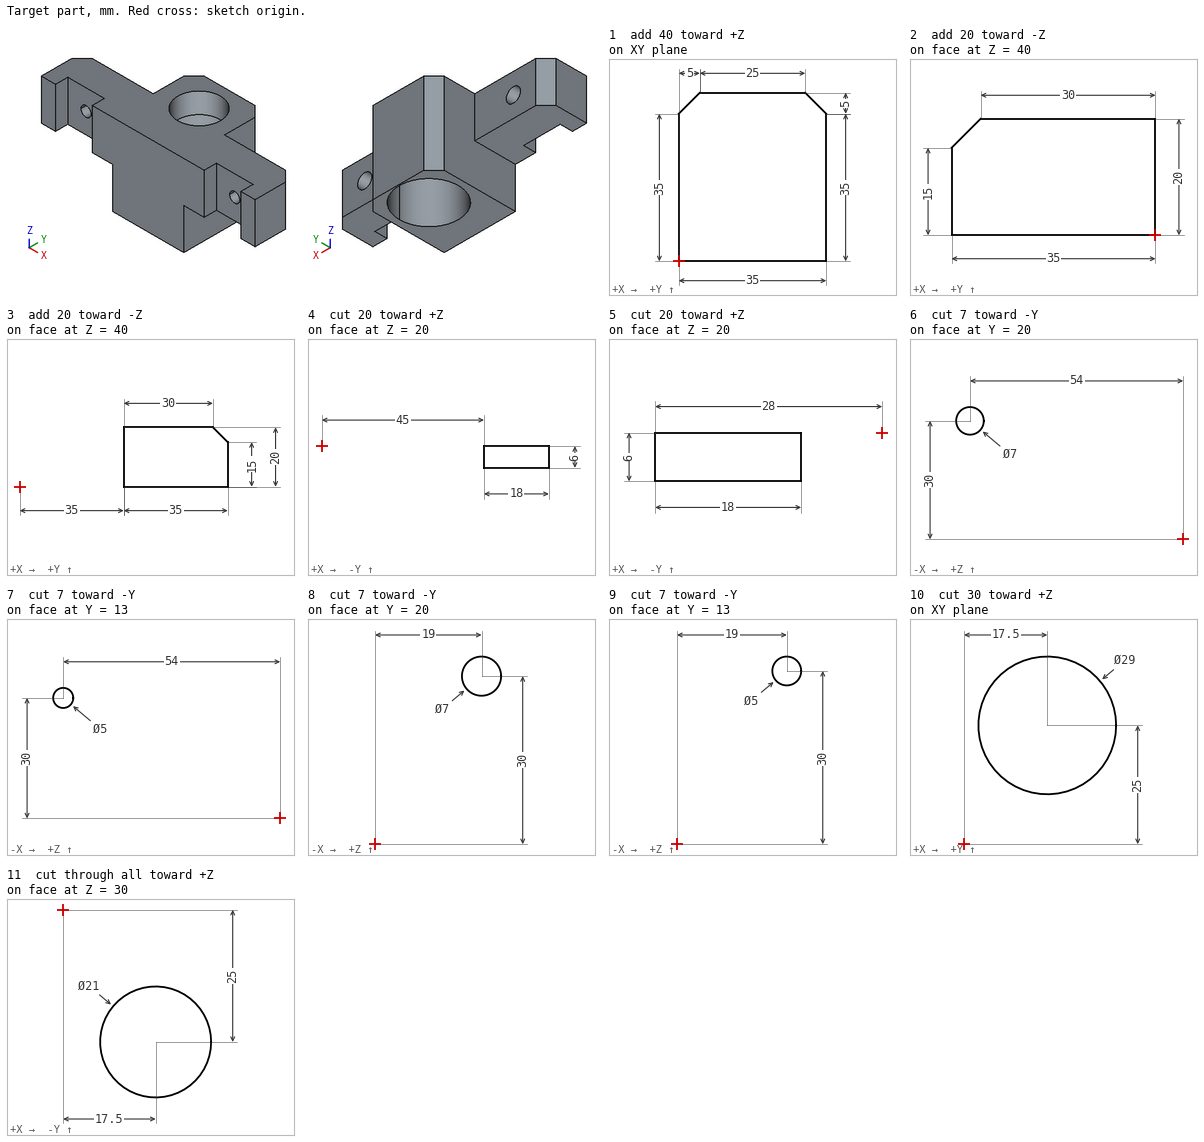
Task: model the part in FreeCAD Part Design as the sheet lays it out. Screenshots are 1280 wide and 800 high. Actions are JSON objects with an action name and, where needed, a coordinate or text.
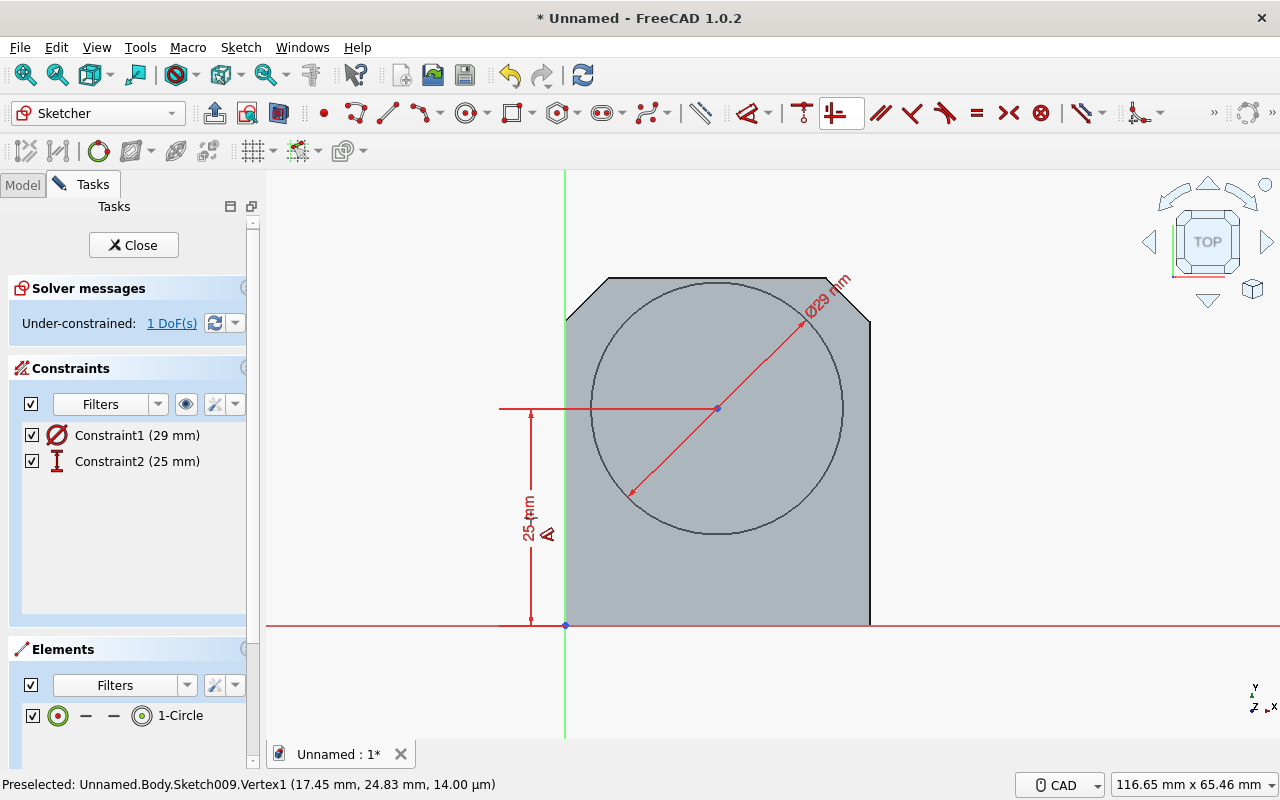
{"action": "left_click", "coordinate": [717, 409]}
{"action": "left_click", "coordinate": [641, 660]}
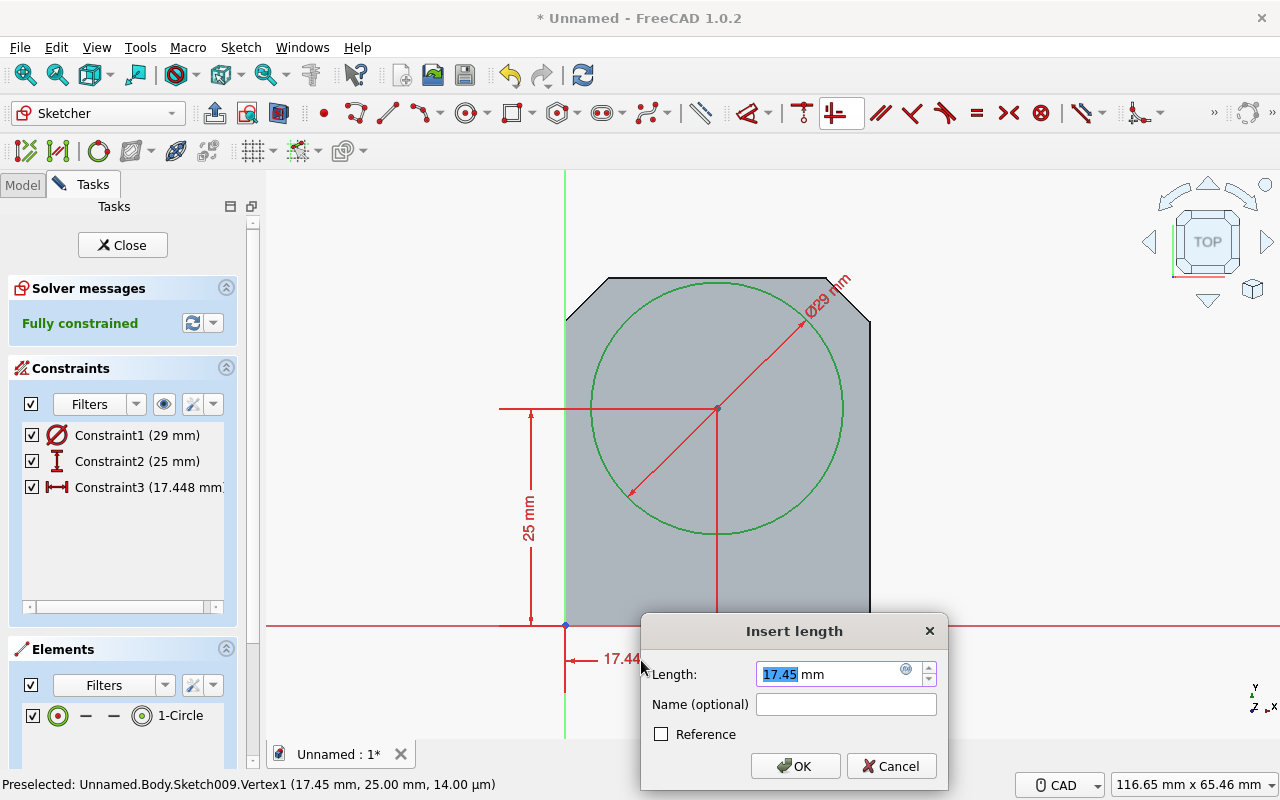
{"action": "type", "text": "17.5"}
{"action": "key", "text": "Return"}
{"action": "key", "text": "Escape"}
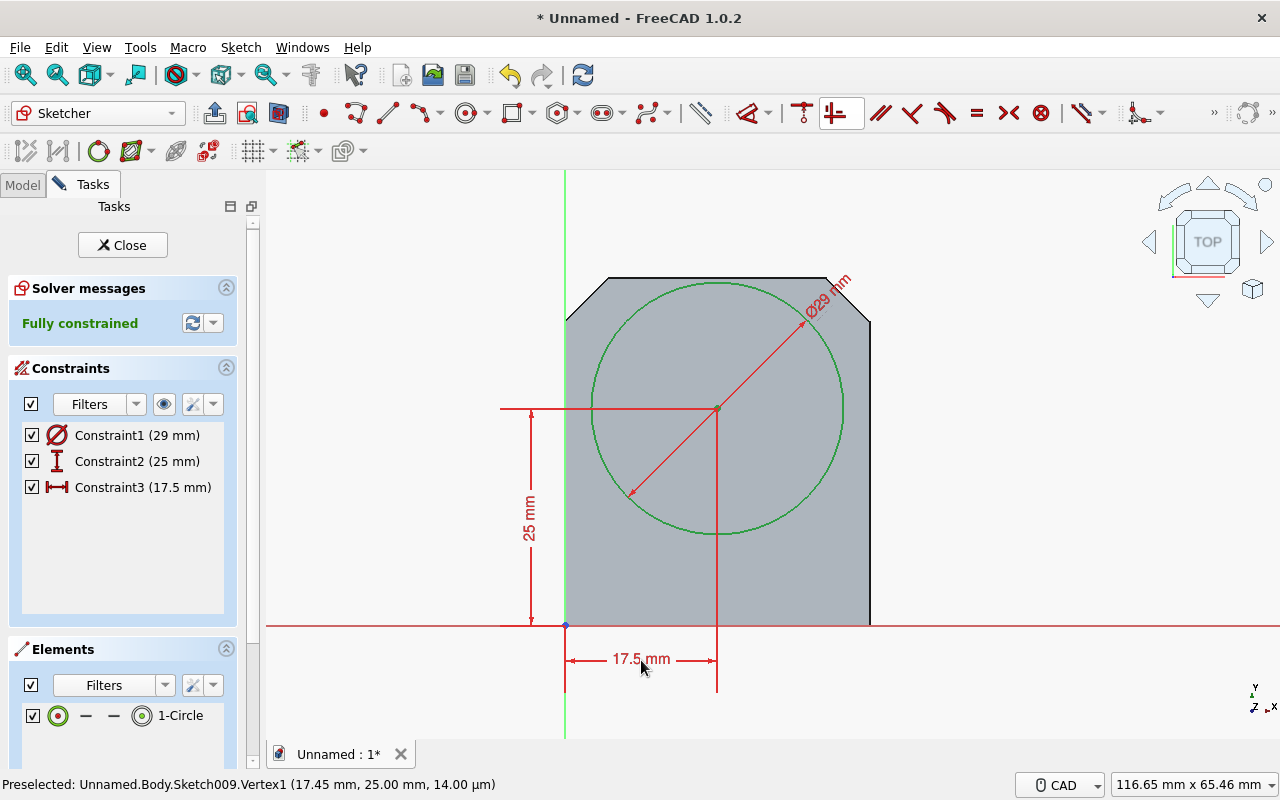
{"action": "left_click", "coordinate": [123, 245]}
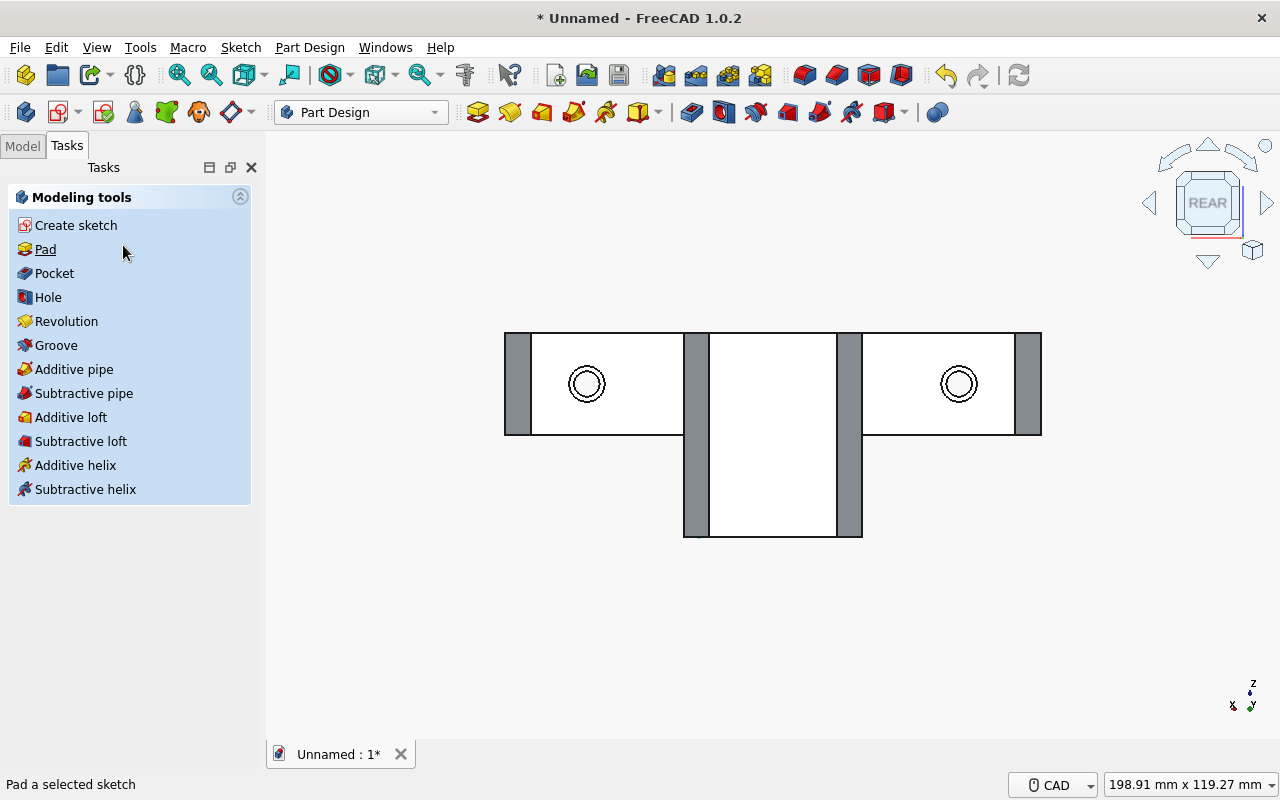
{"action": "left_click", "coordinate": [692, 112]}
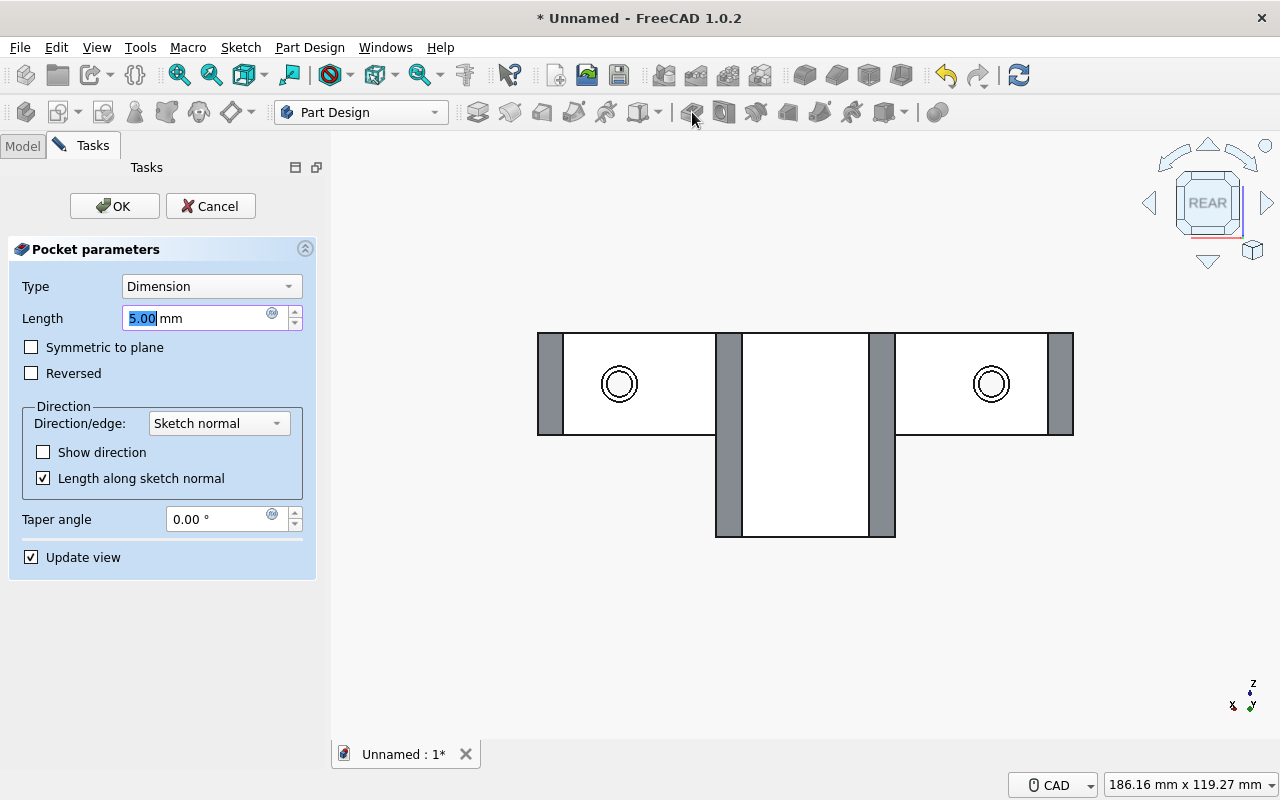
{"action": "type", "text": "30"}
{"action": "key", "text": "Tab"}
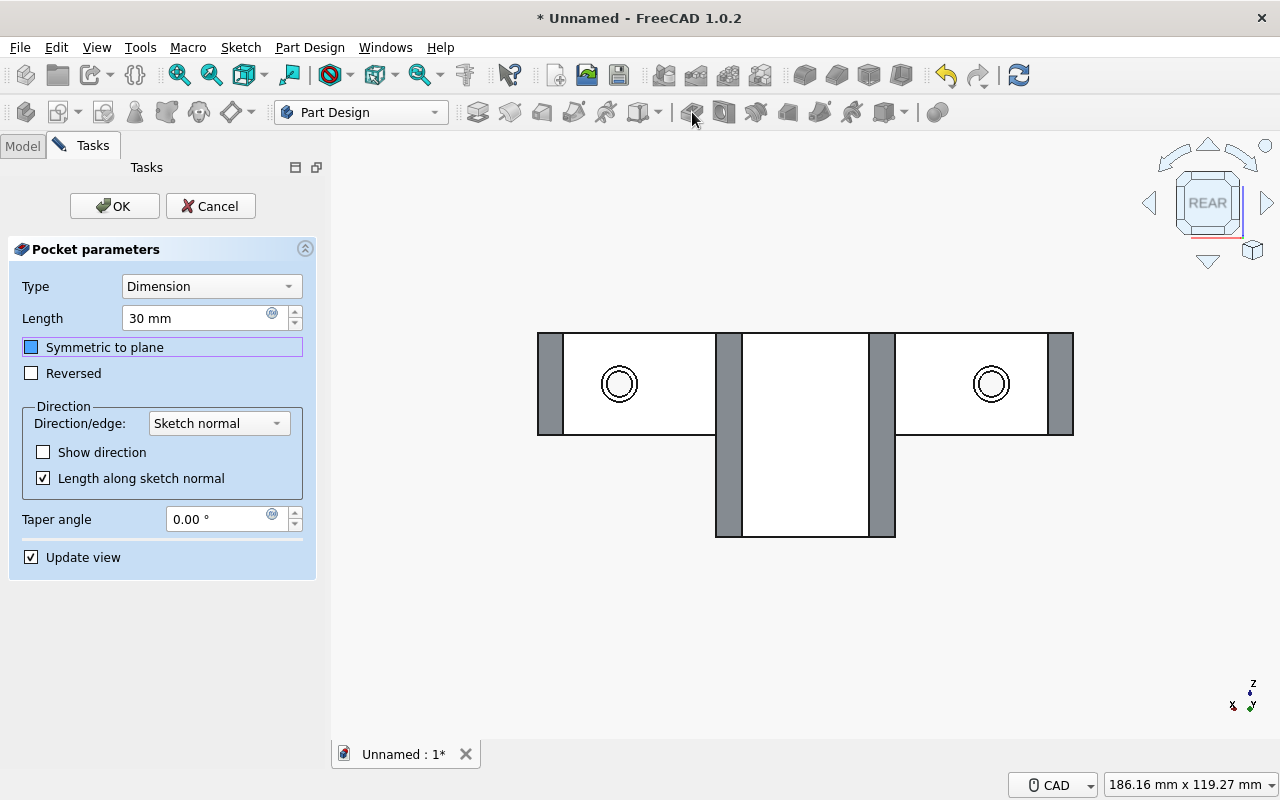
{"action": "left_click", "coordinate": [30, 373]}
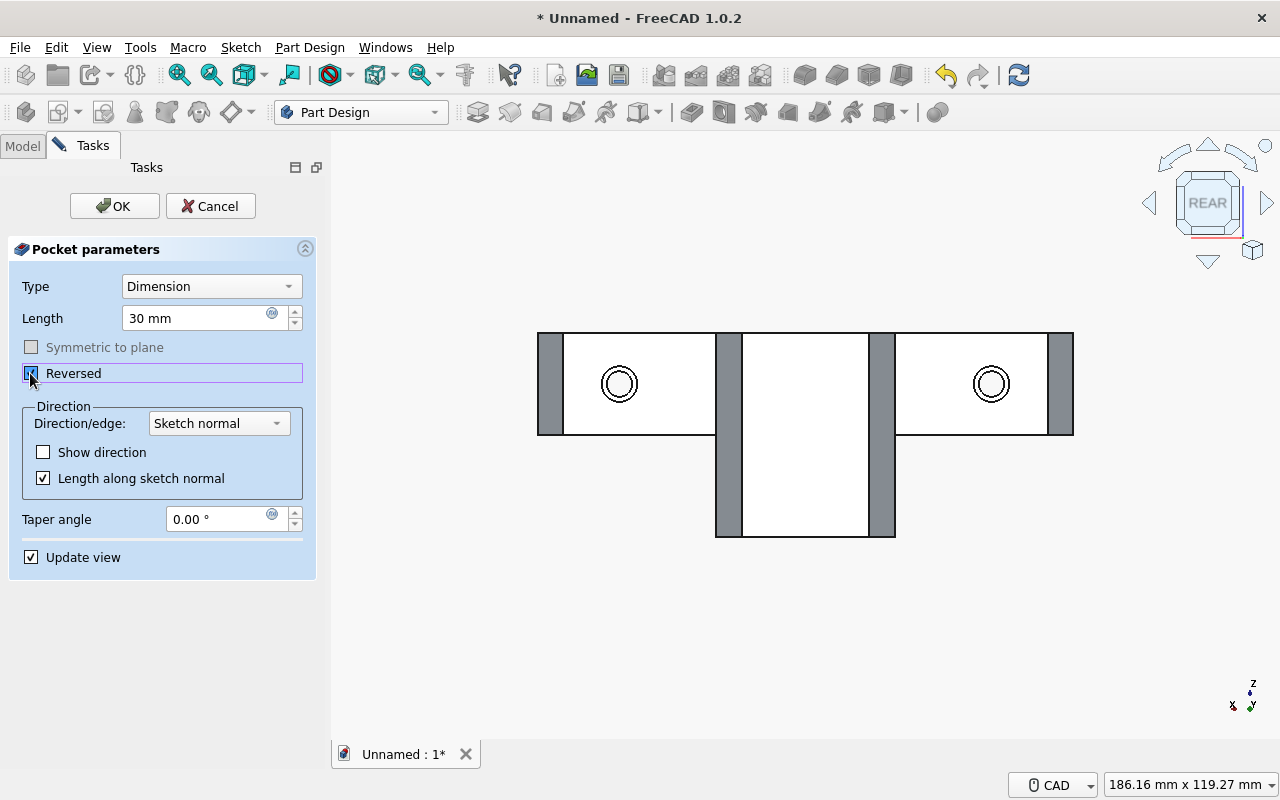
{"action": "left_click", "coordinate": [115, 206]}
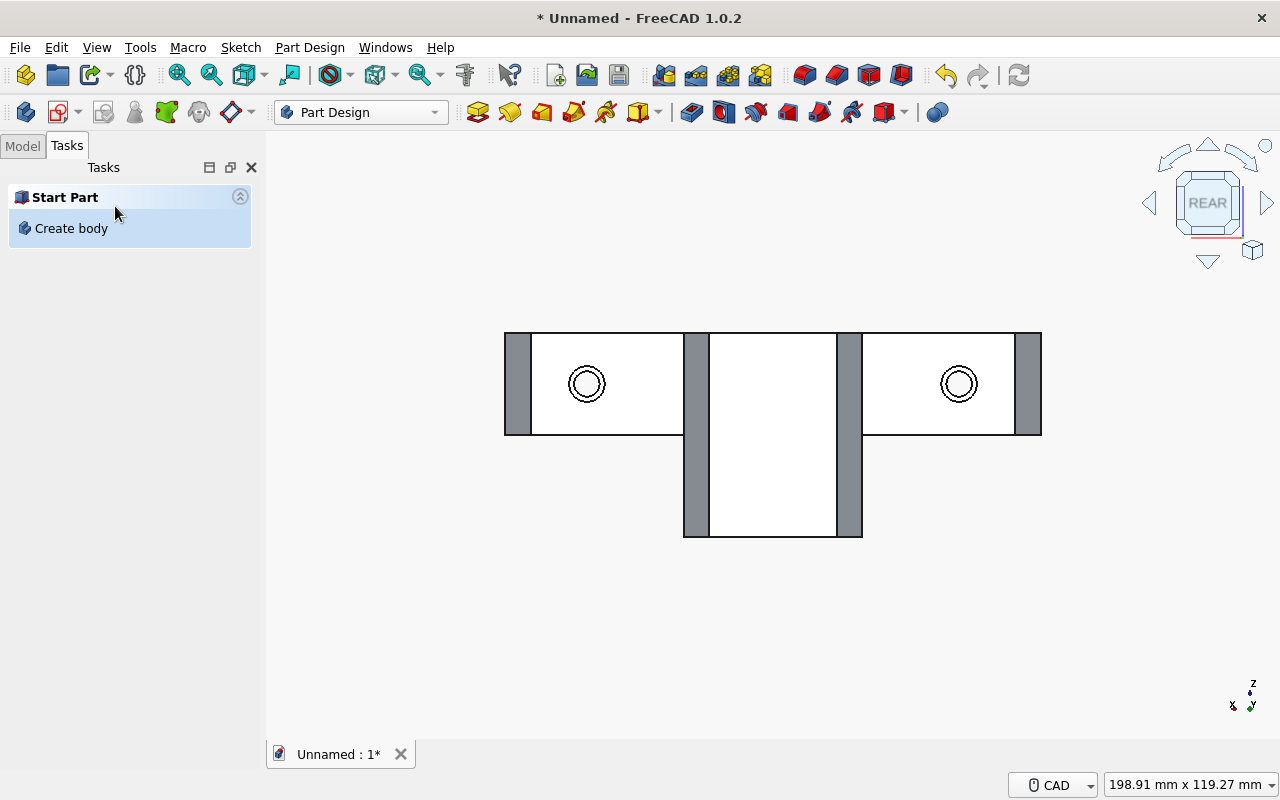
{"action": "key", "text": "5"}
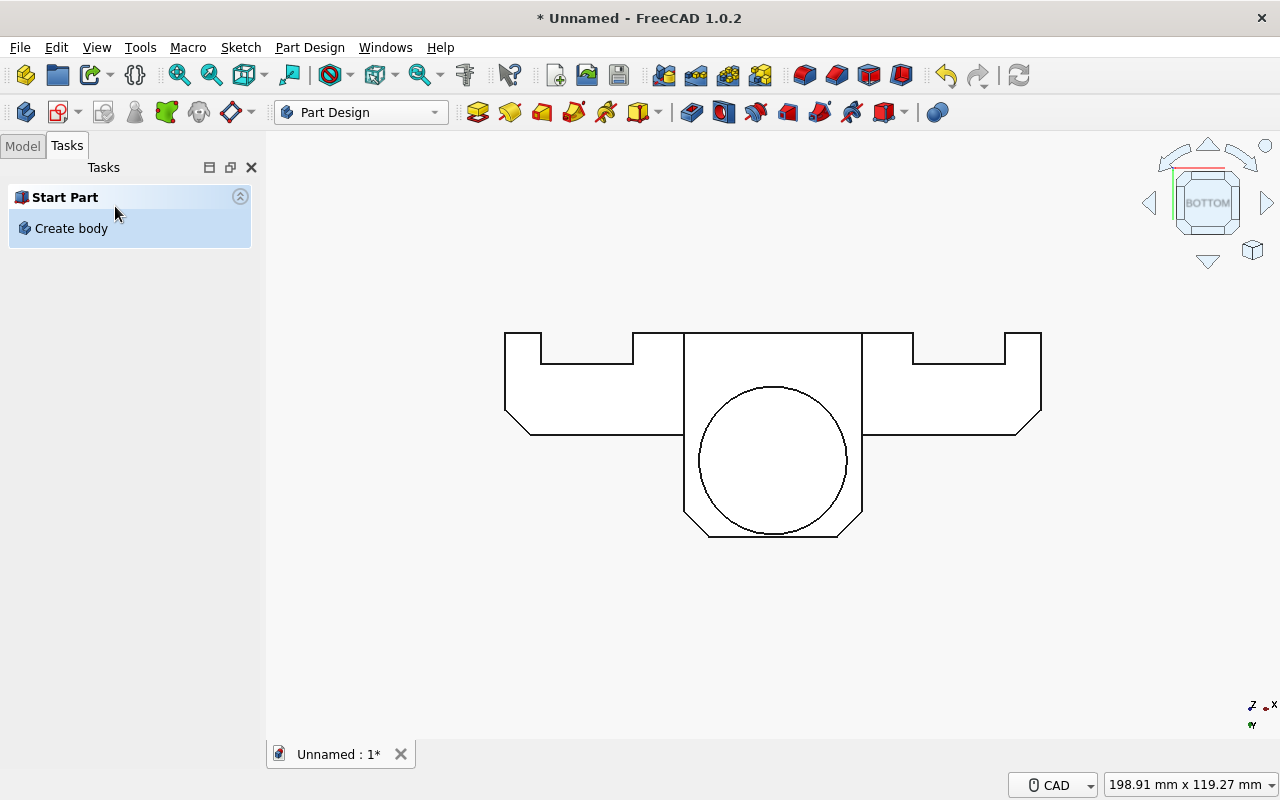
{"action": "left_click", "coordinate": [773, 459]}